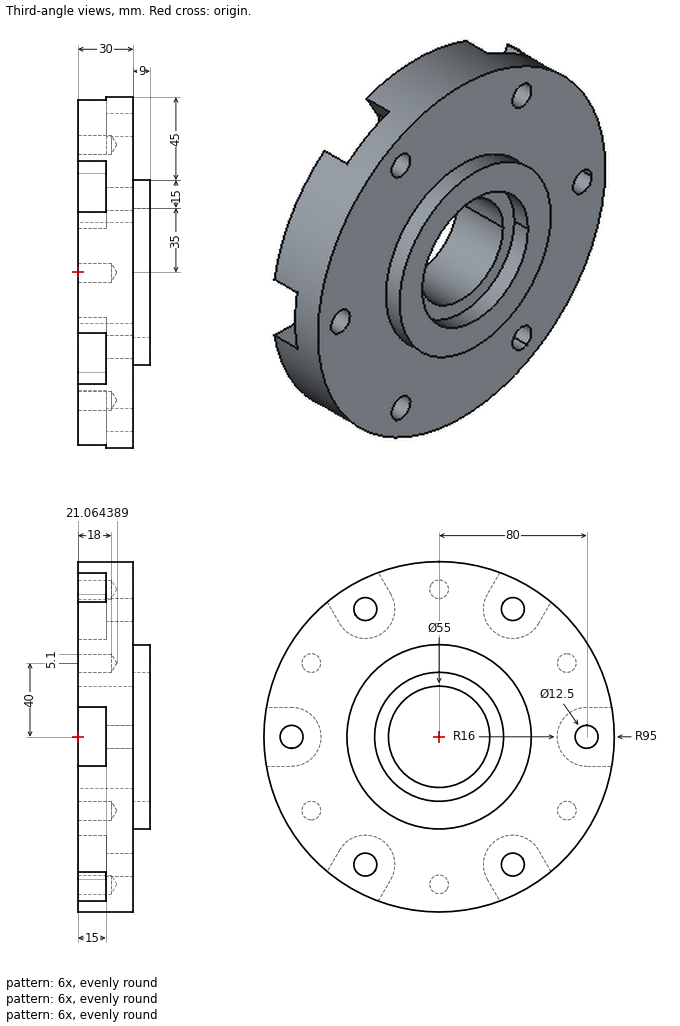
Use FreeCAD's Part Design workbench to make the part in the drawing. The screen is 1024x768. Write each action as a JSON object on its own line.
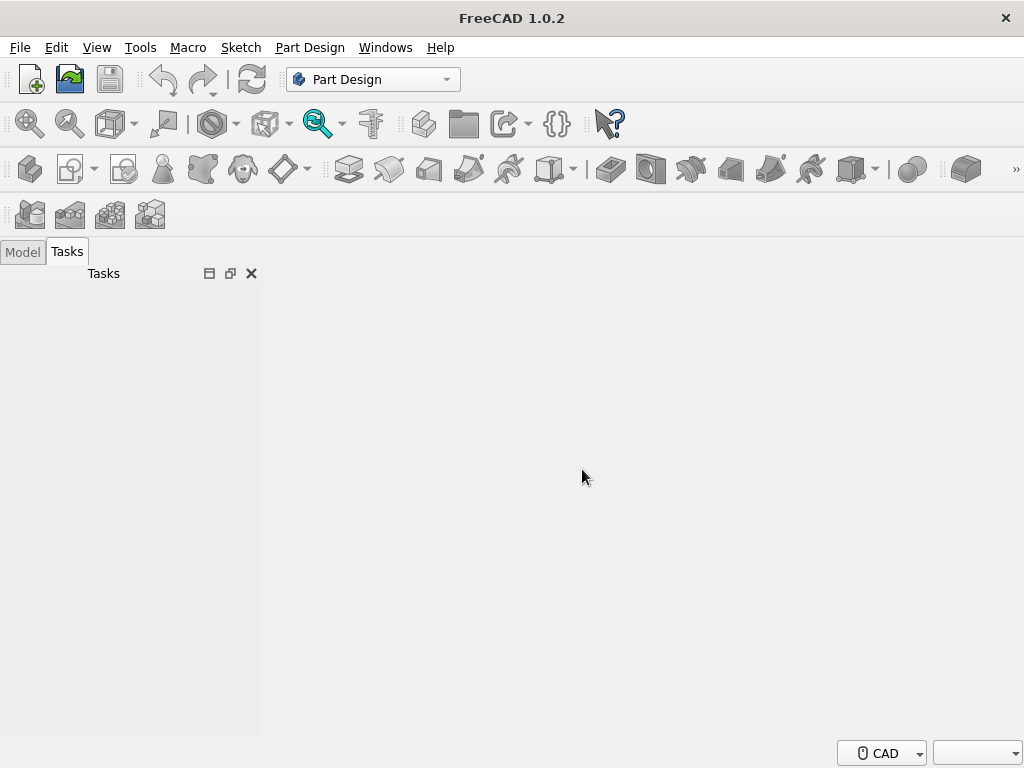
{"action": "left_click", "coordinate": [30, 80]}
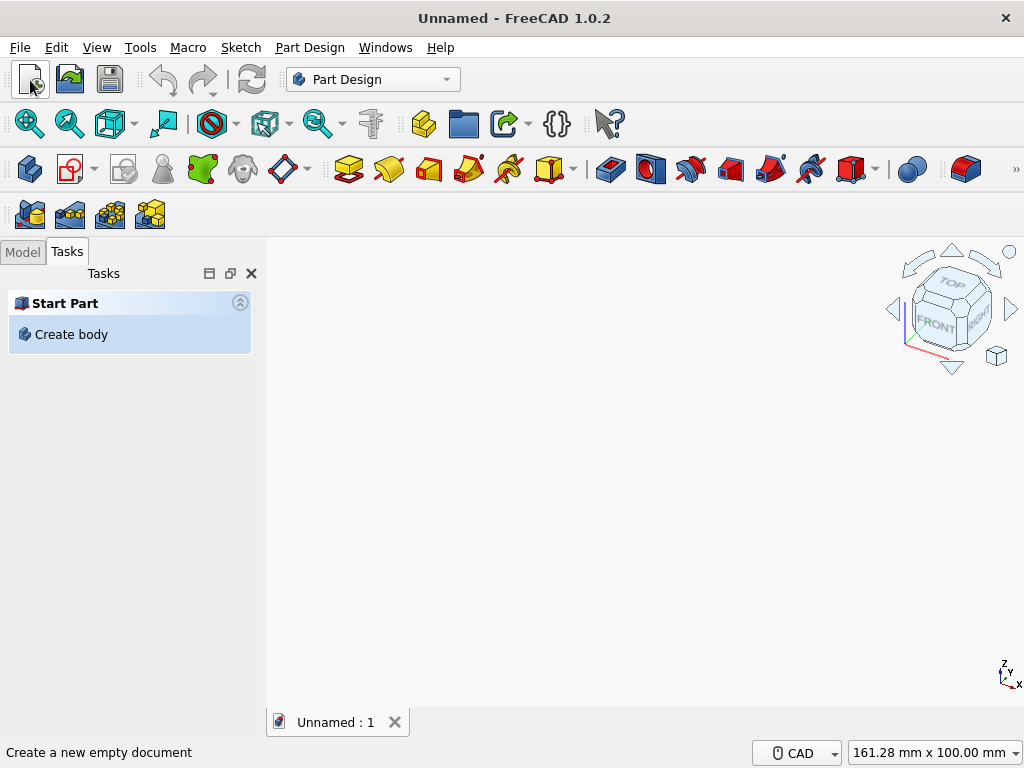
{"action": "left_click", "coordinate": [70, 170]}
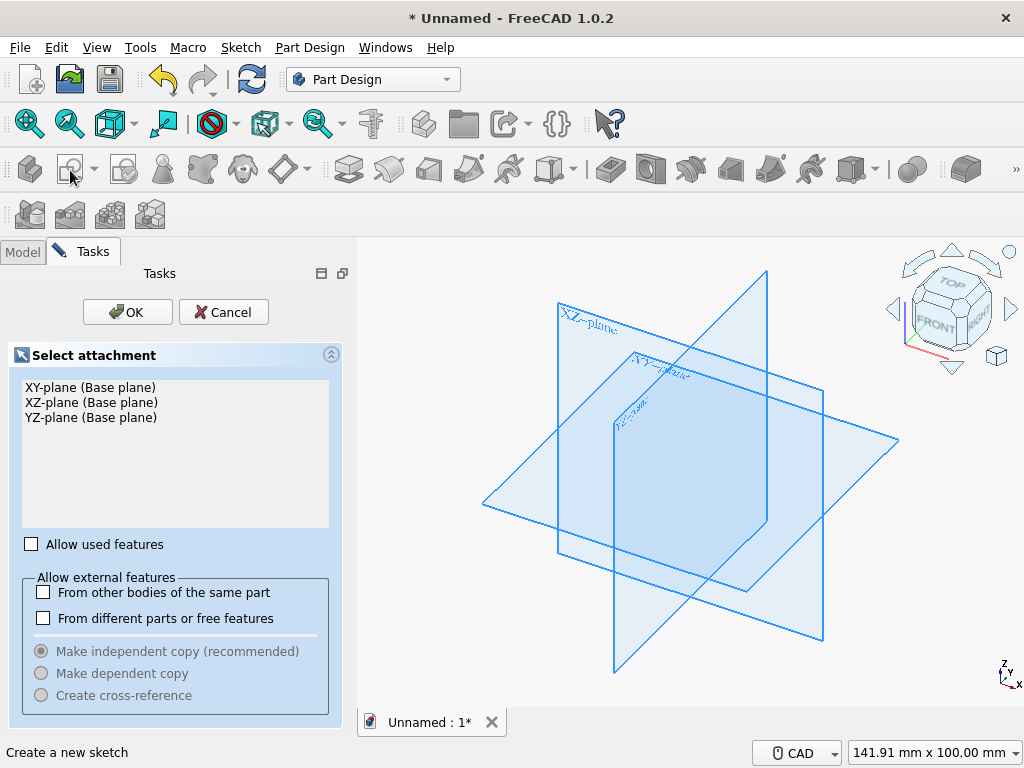
{"action": "left_click", "coordinate": [82, 388]}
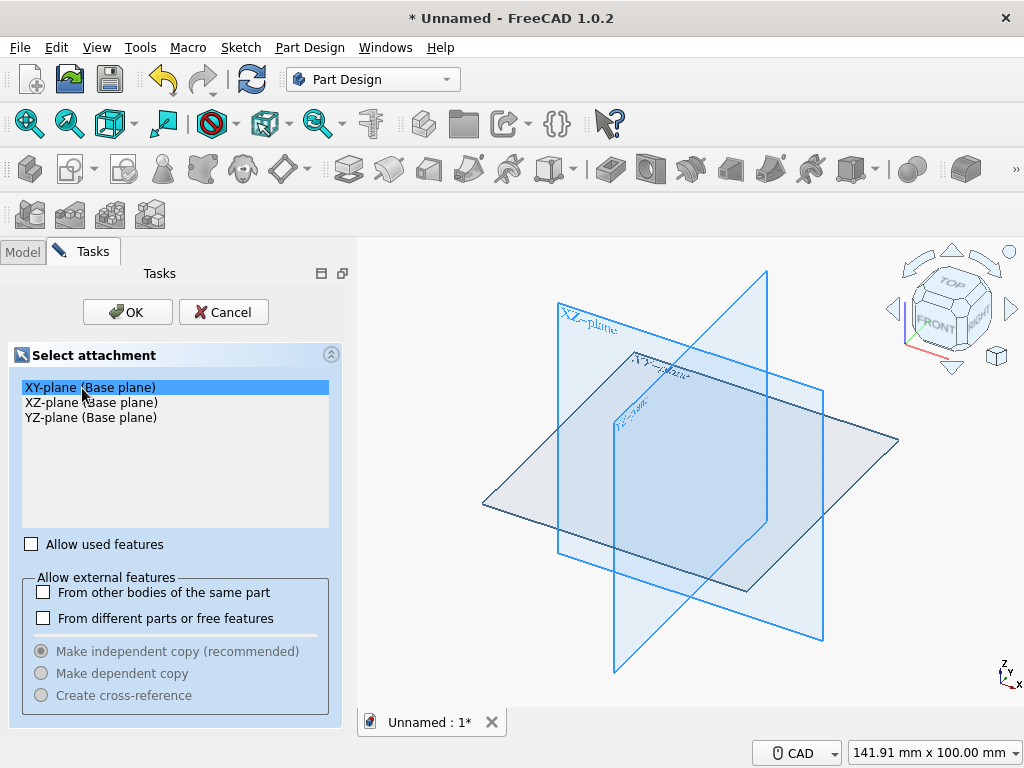
{"action": "left_click", "coordinate": [128, 312]}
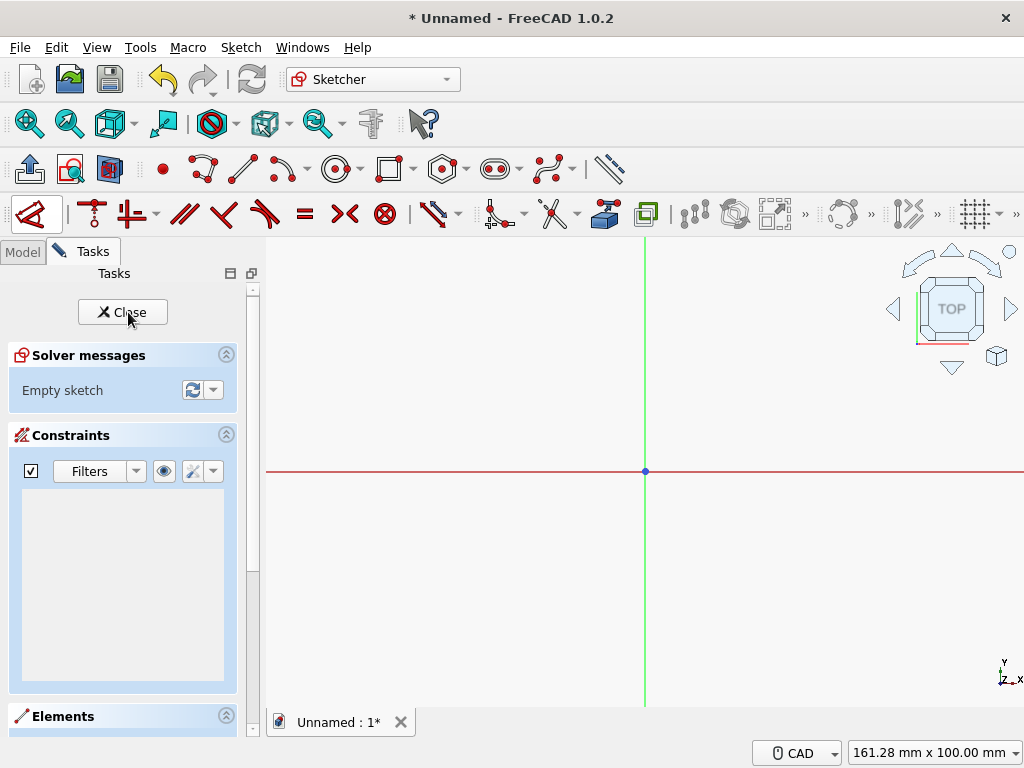
{"action": "scroll", "coordinate": [382, 679], "scroll_direction": "down", "scroll_amount": 3}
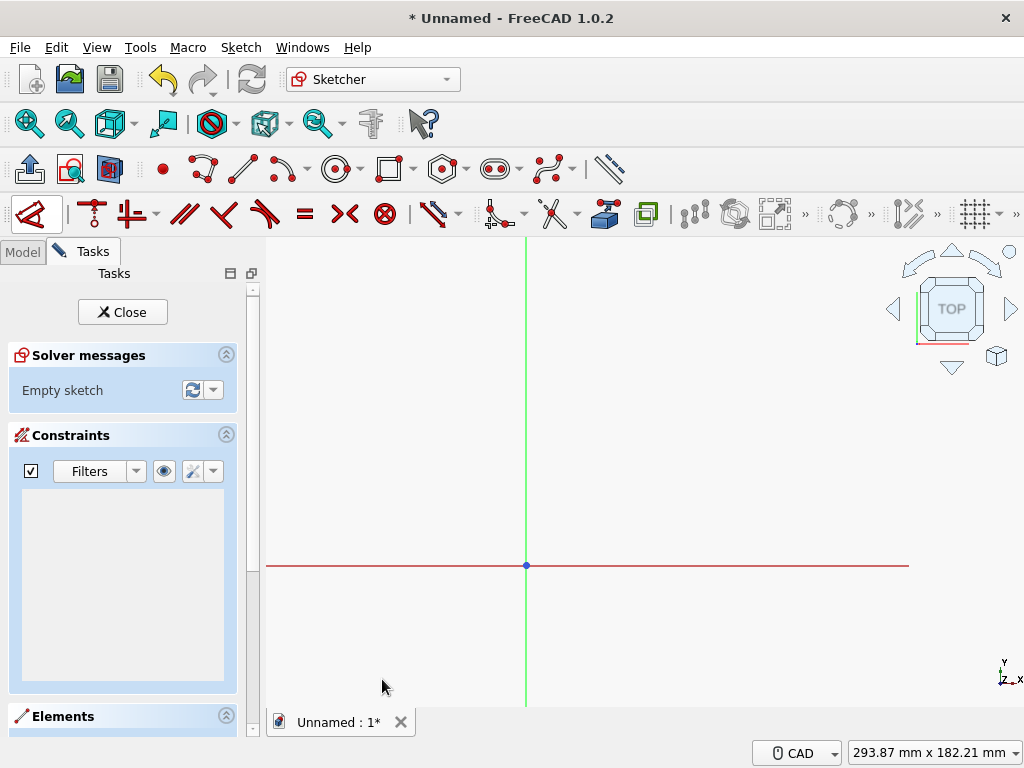
{"action": "left_click", "coordinate": [204, 170]}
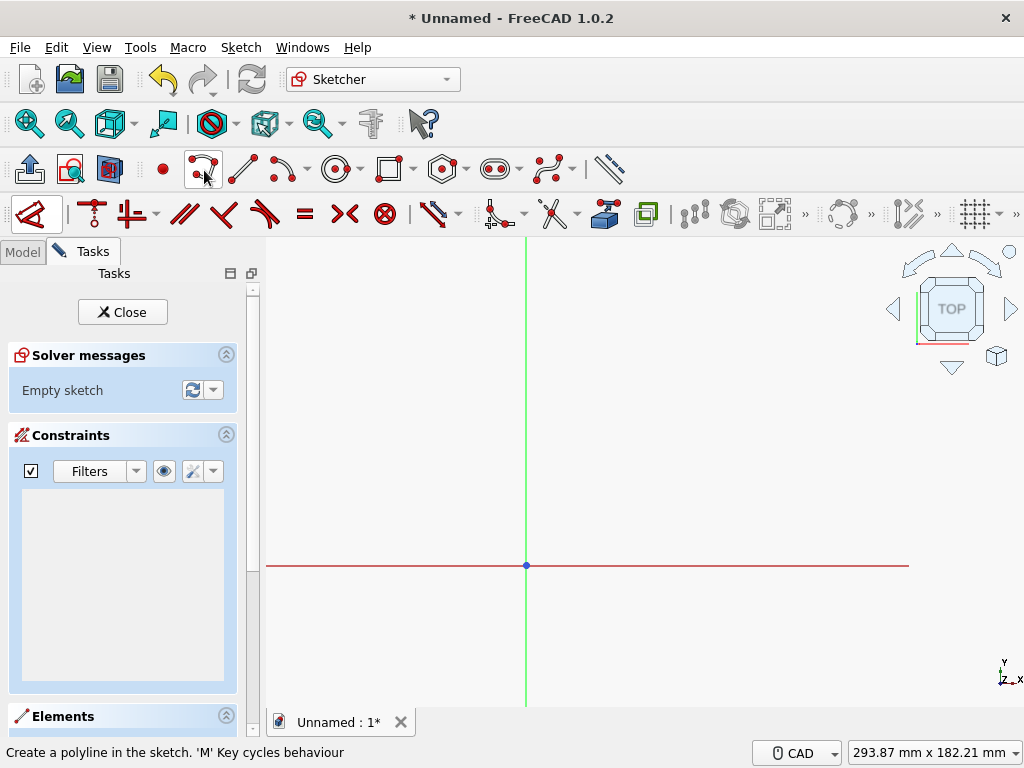
{"action": "left_click", "coordinate": [526, 566]}
{"action": "left_click", "coordinate": [604, 557]}
{"action": "left_click", "coordinate": [604, 476]}
{"action": "left_click", "coordinate": [627, 476]}
{"action": "left_click", "coordinate": [627, 437]}
{"action": "left_click", "coordinate": [604, 437]}
{"action": "left_click", "coordinate": [604, 321]}
{"action": "left_click", "coordinate": [535, 321]}
{"action": "left_click", "coordinate": [526, 566]}
{"action": "key", "text": "Escape"}
{"action": "key", "text": "Escape"}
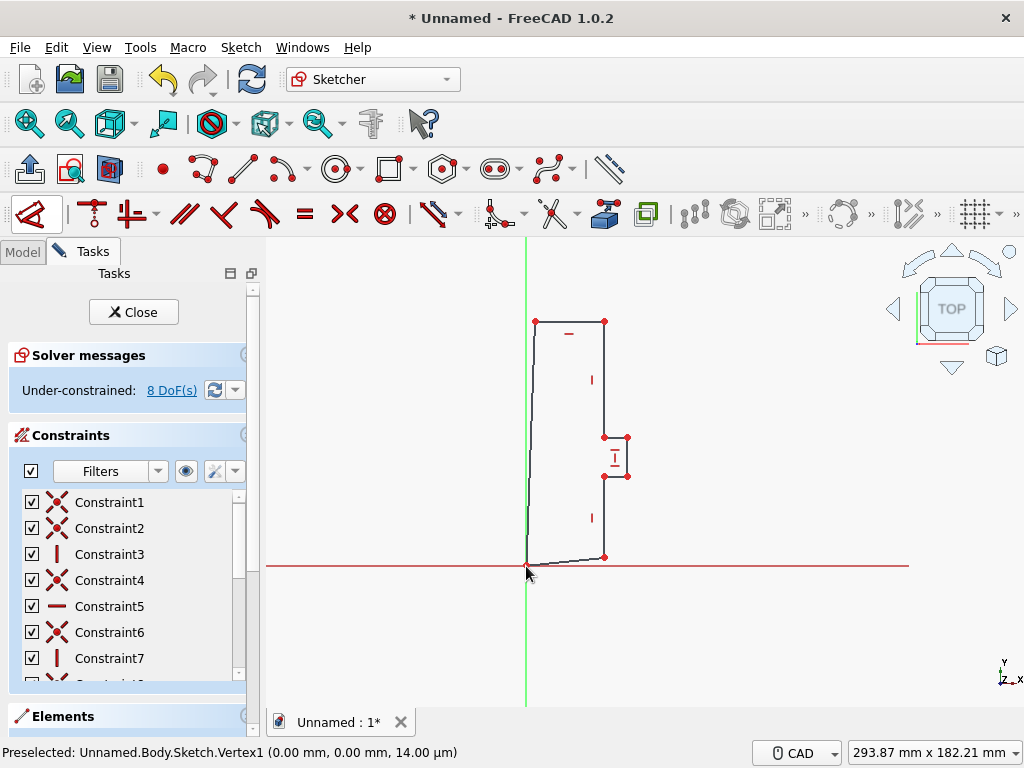
{"action": "left_click", "coordinate": [550, 563]}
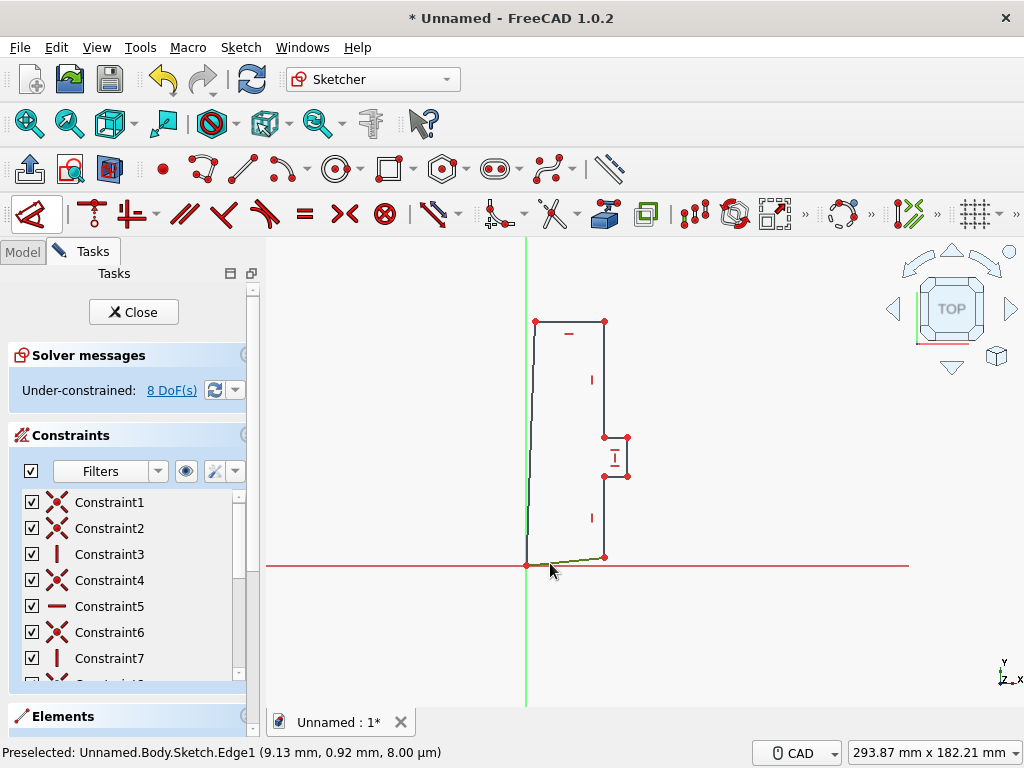
{"action": "key", "text": "h"}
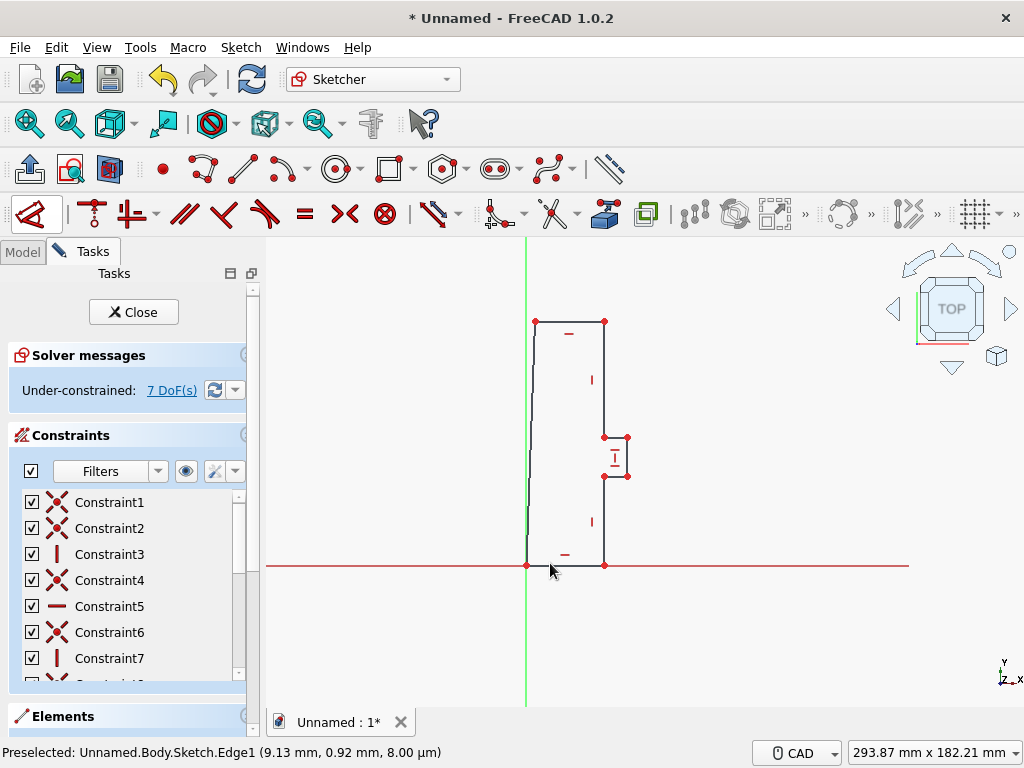
{"action": "left_click", "coordinate": [529, 493]}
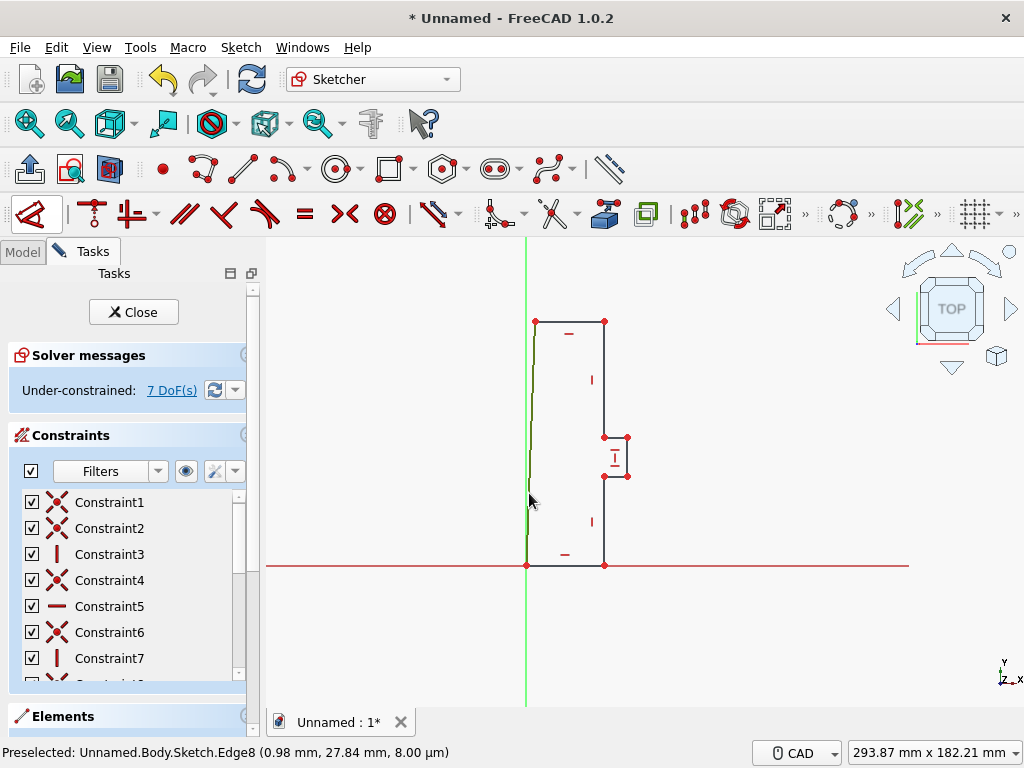
{"action": "key", "text": "v"}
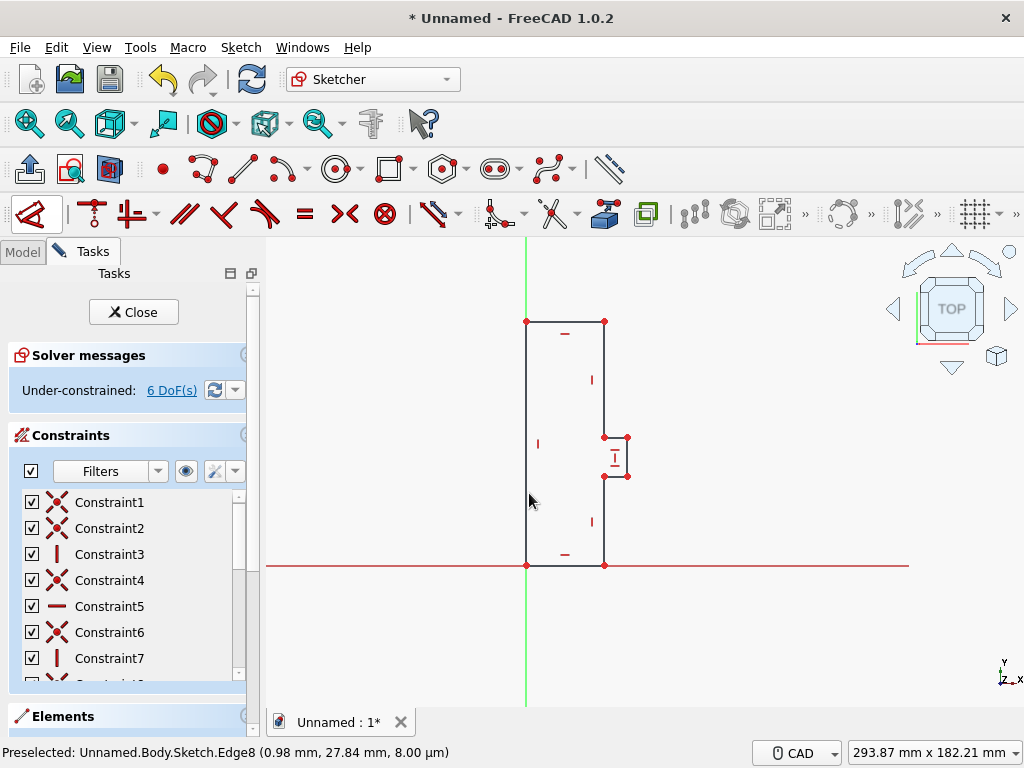
{"action": "left_click", "coordinate": [30, 214]}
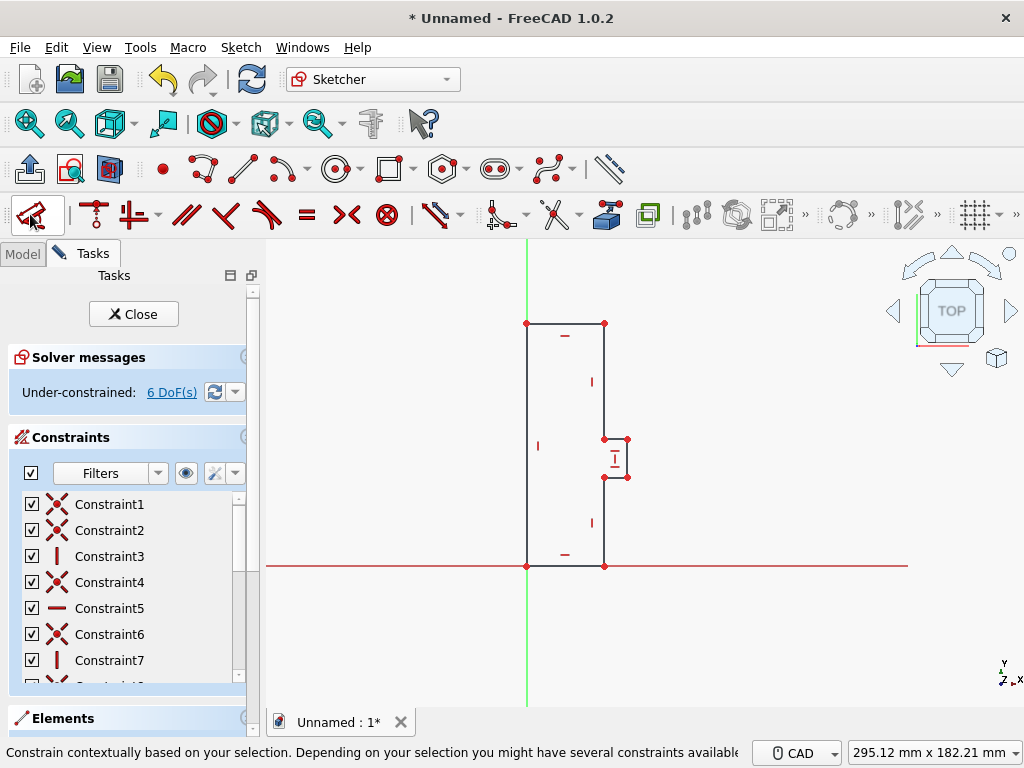
{"action": "scroll", "coordinate": [613, 478], "scroll_direction": "up", "scroll_amount": 3}